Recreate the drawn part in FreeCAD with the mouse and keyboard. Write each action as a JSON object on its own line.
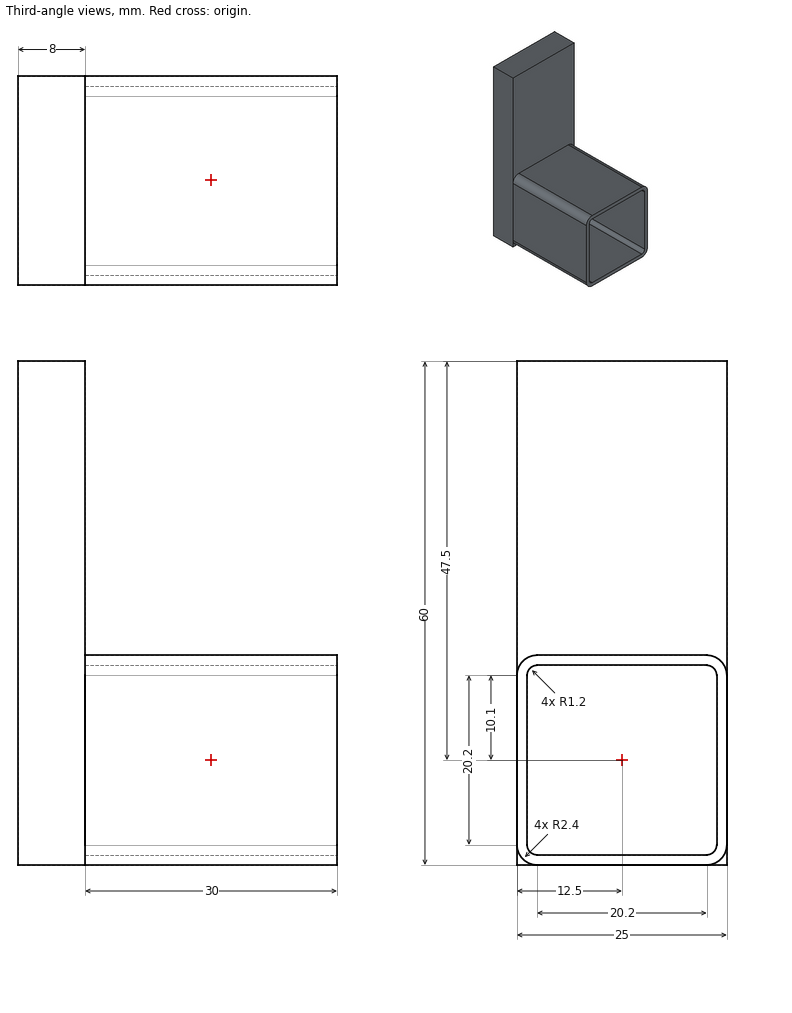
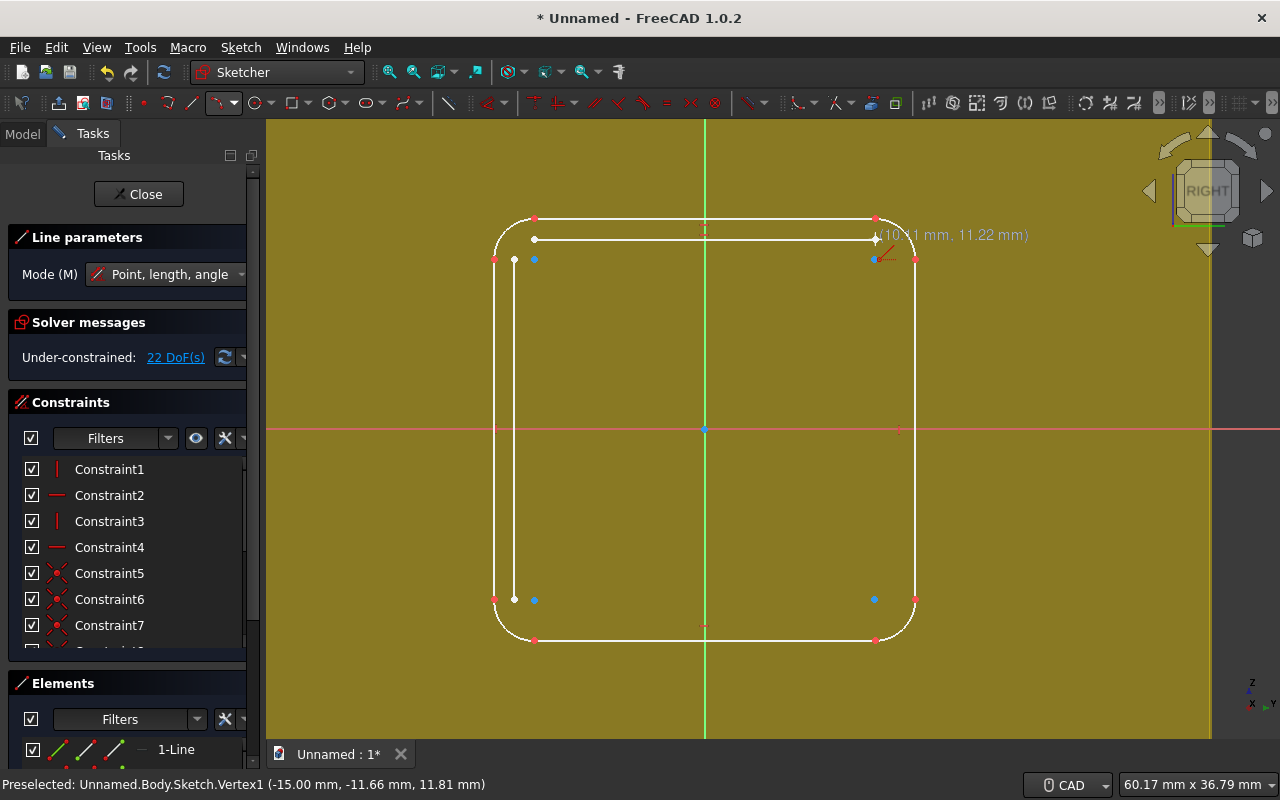
{"action": "left_click", "coordinate": [895, 259]}
{"action": "left_click", "coordinate": [895, 599]}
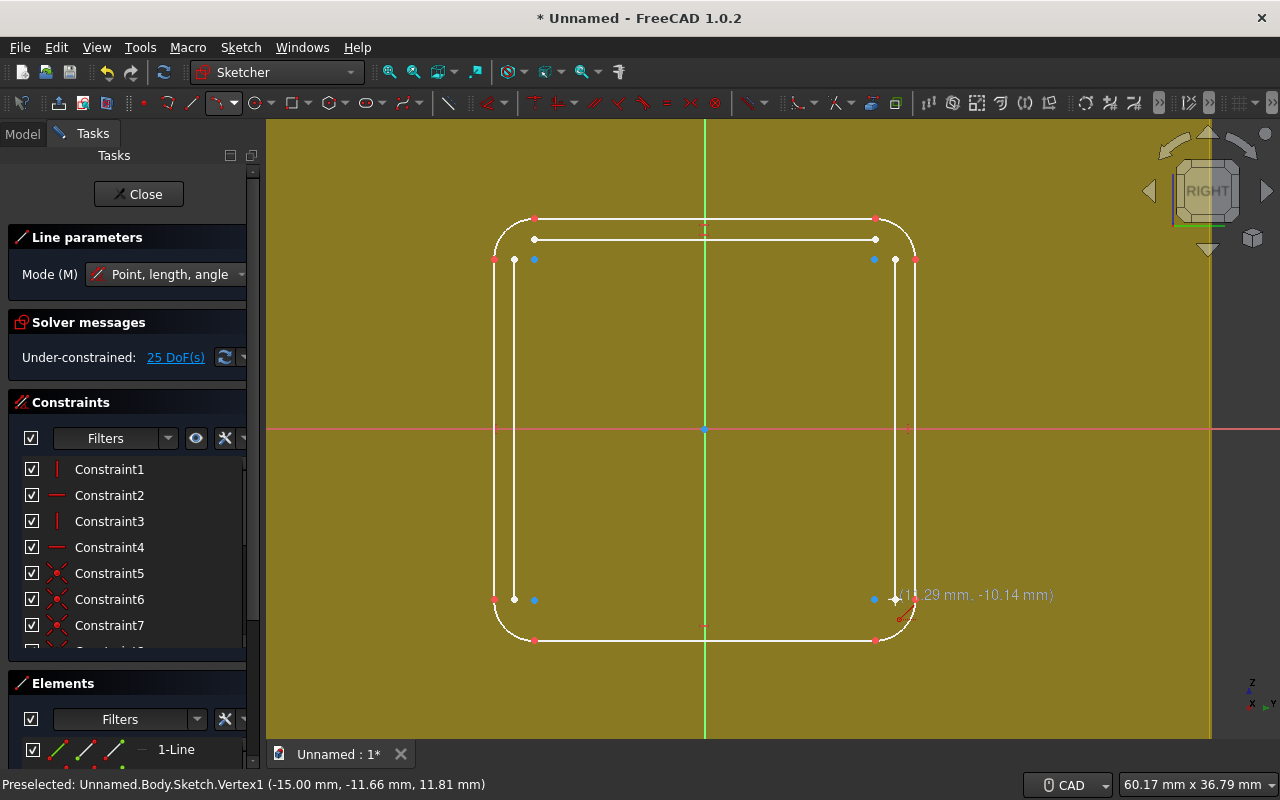
{"action": "left_click", "coordinate": [875, 620]}
{"action": "left_click", "coordinate": [534, 620]}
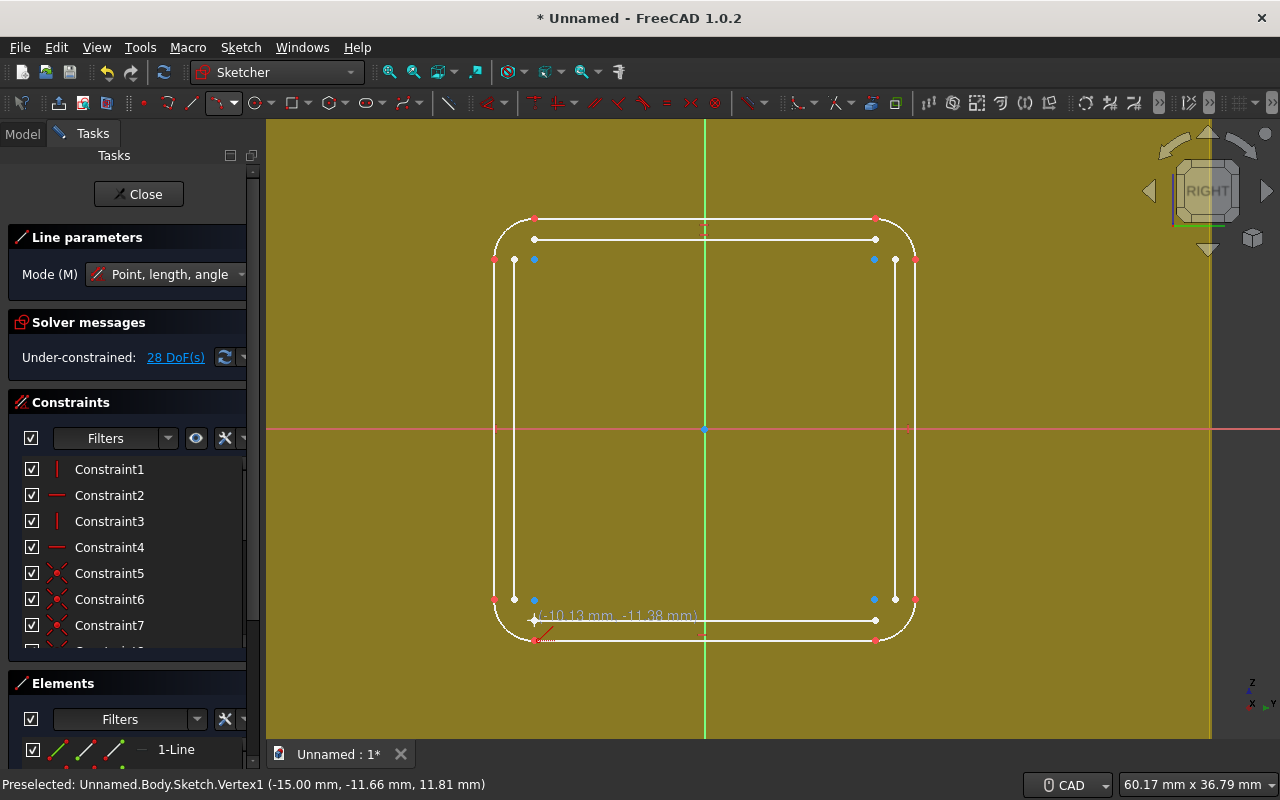
{"action": "key", "text": "g 3 a"}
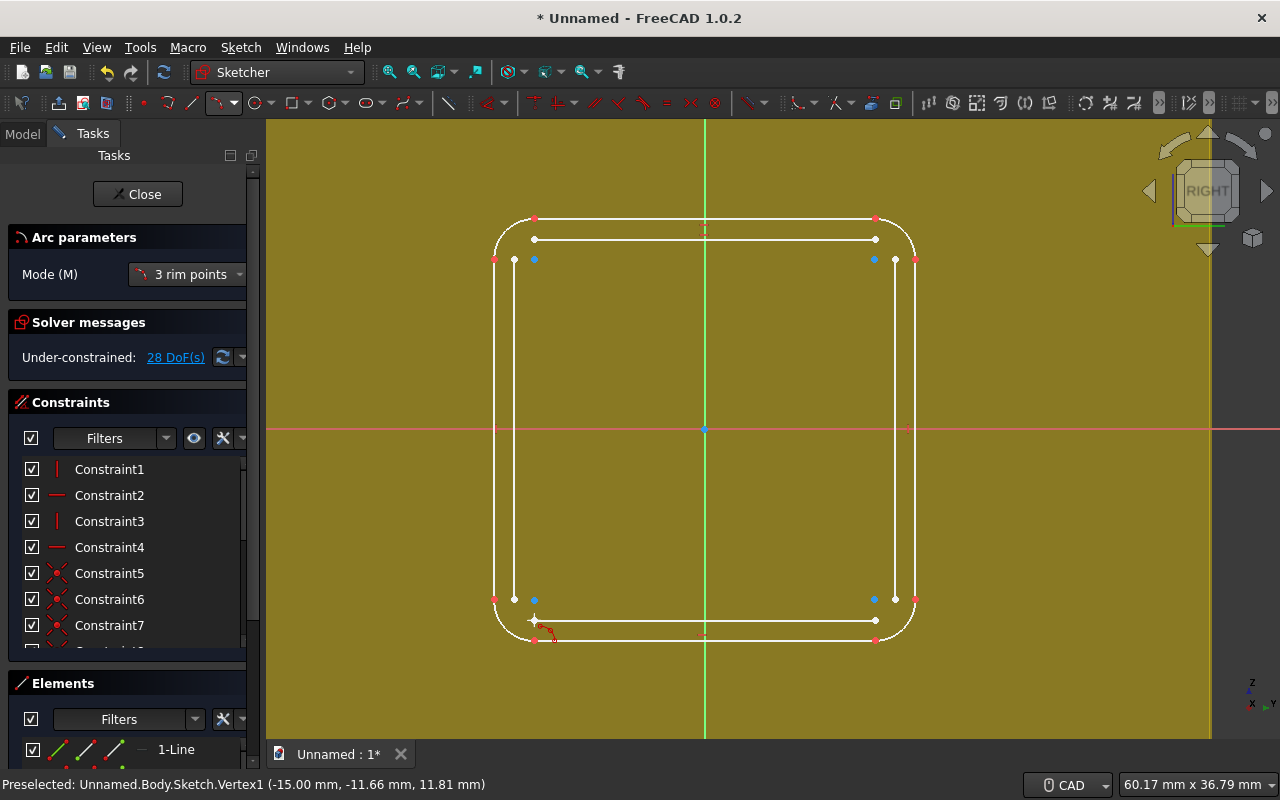
{"action": "left_click", "coordinate": [514, 260]}
{"action": "left_click", "coordinate": [534, 240]}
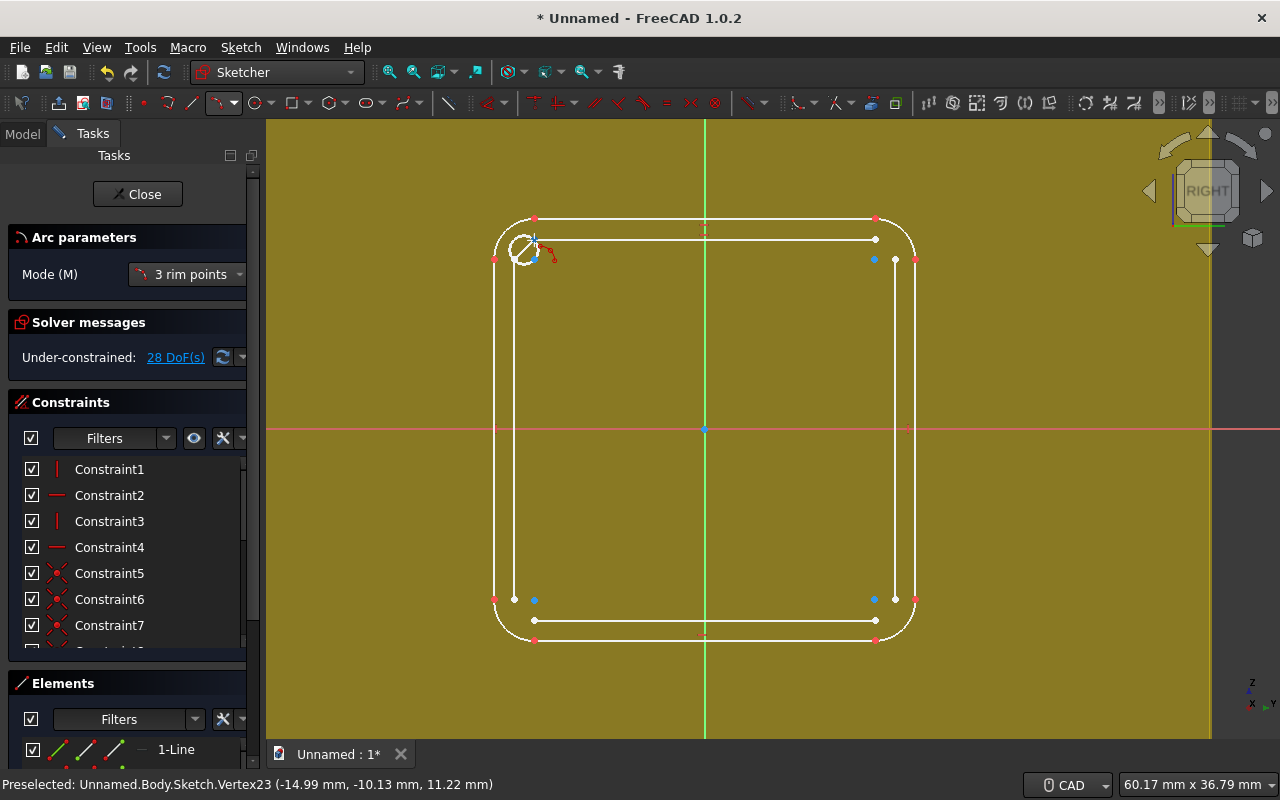
{"action": "scroll", "coordinate": [520, 245], "scroll_direction": "up", "scroll_amount": 5}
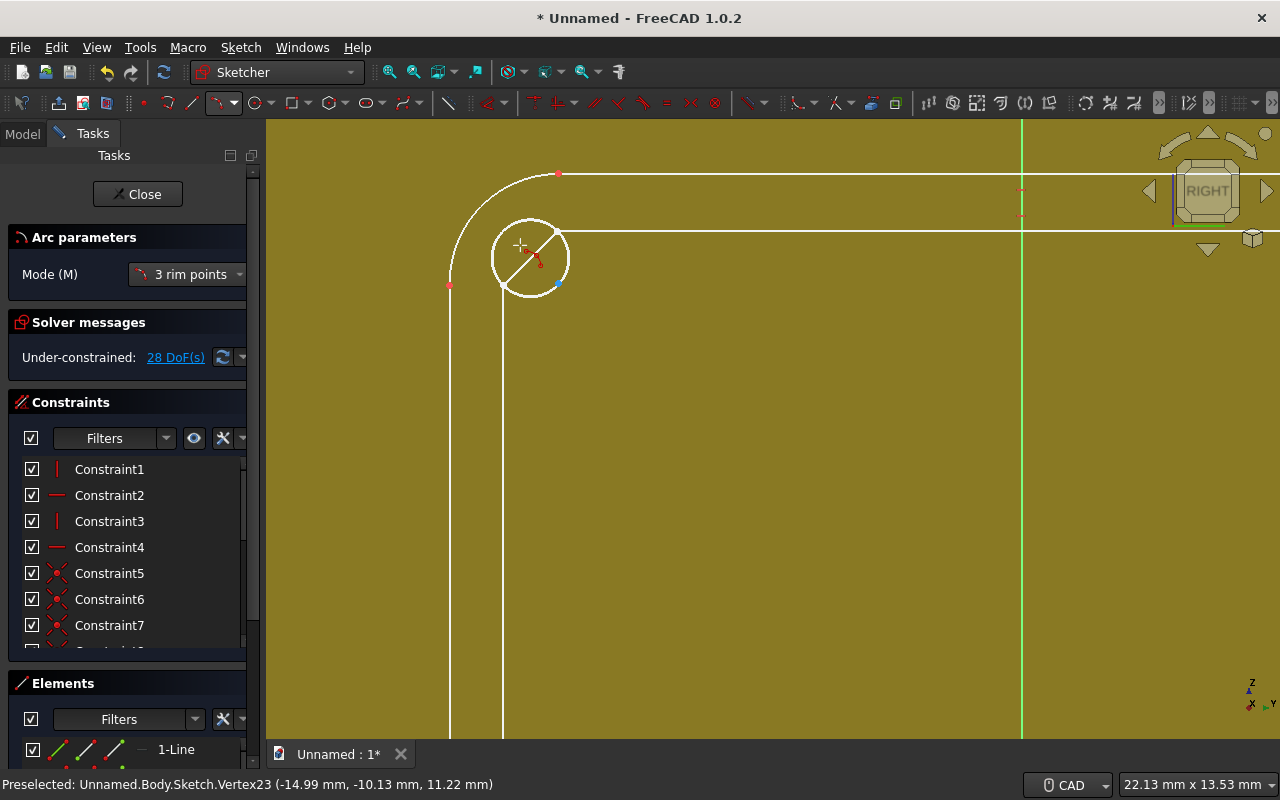
{"action": "left_click", "coordinate": [520, 244]}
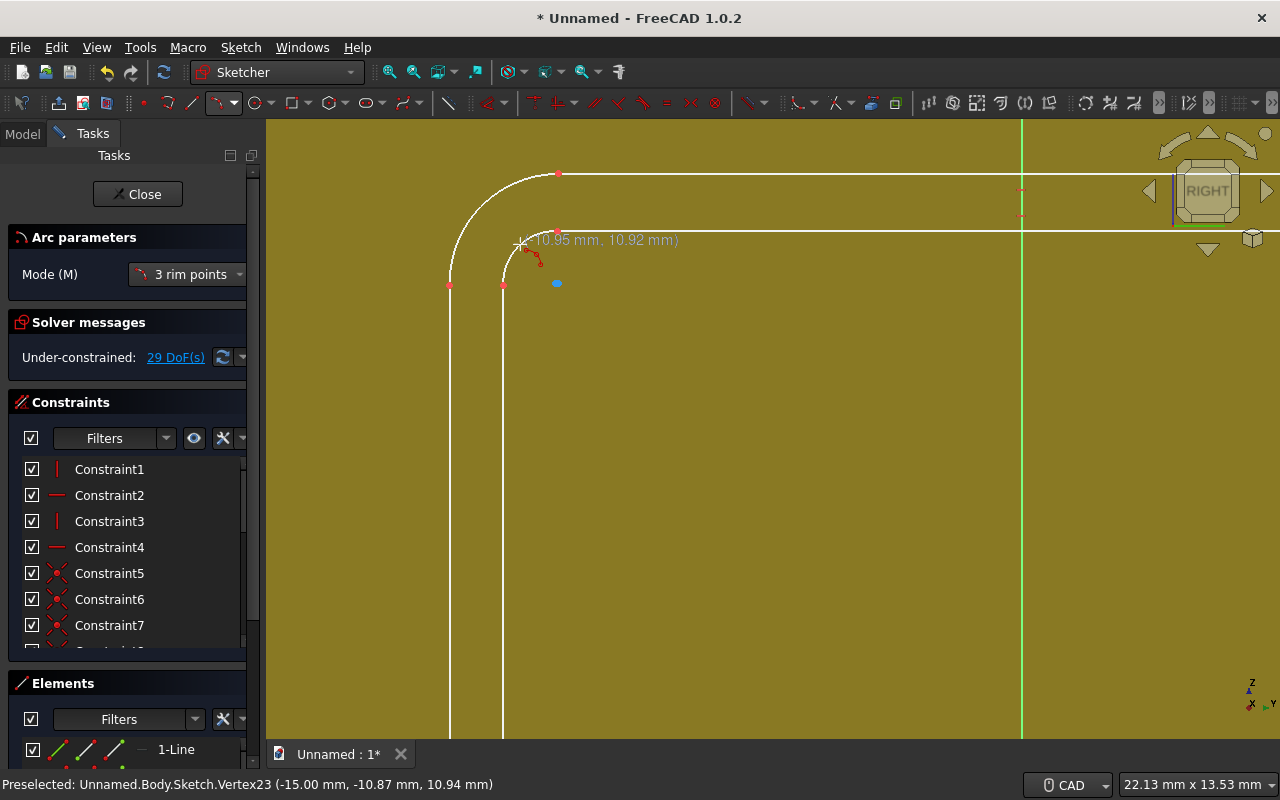
{"action": "scroll", "coordinate": [520, 245], "scroll_direction": "down", "scroll_amount": 5}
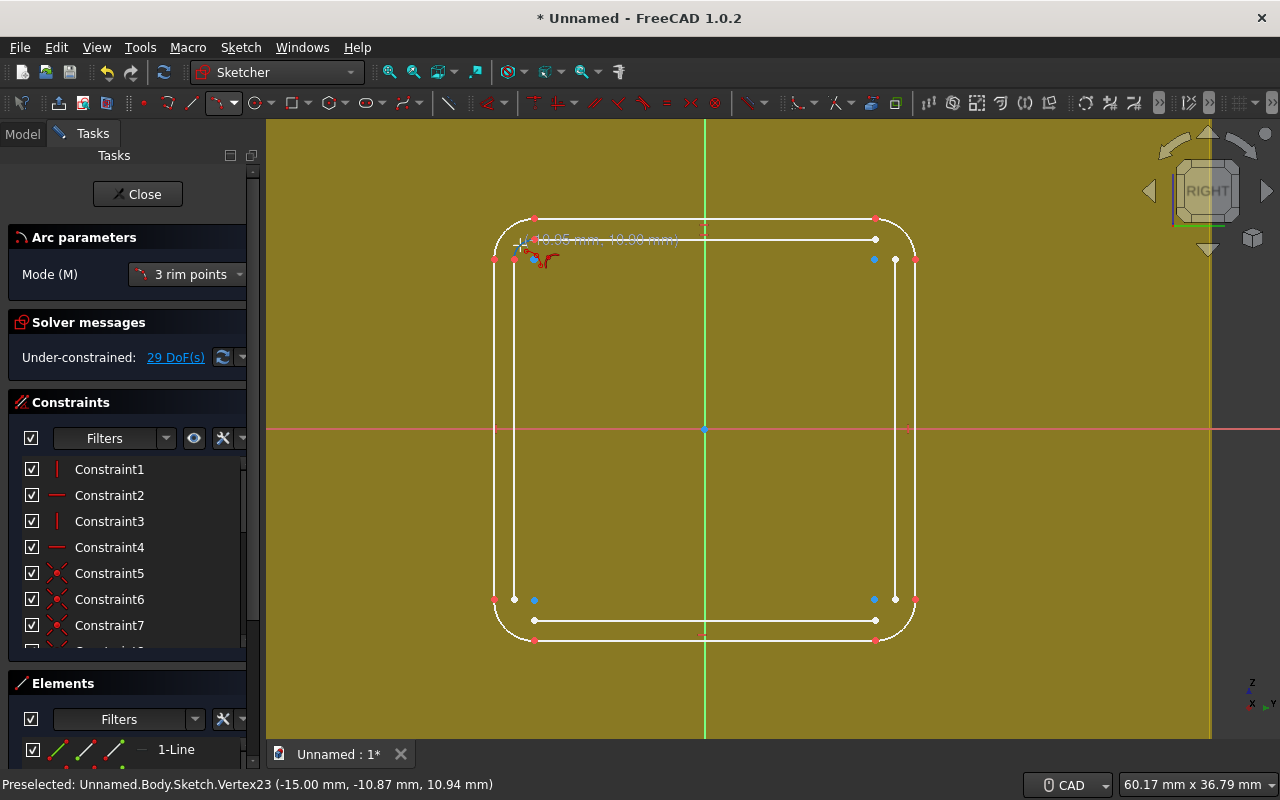
{"action": "left_click", "coordinate": [875, 240]}
{"action": "left_click", "coordinate": [895, 260]}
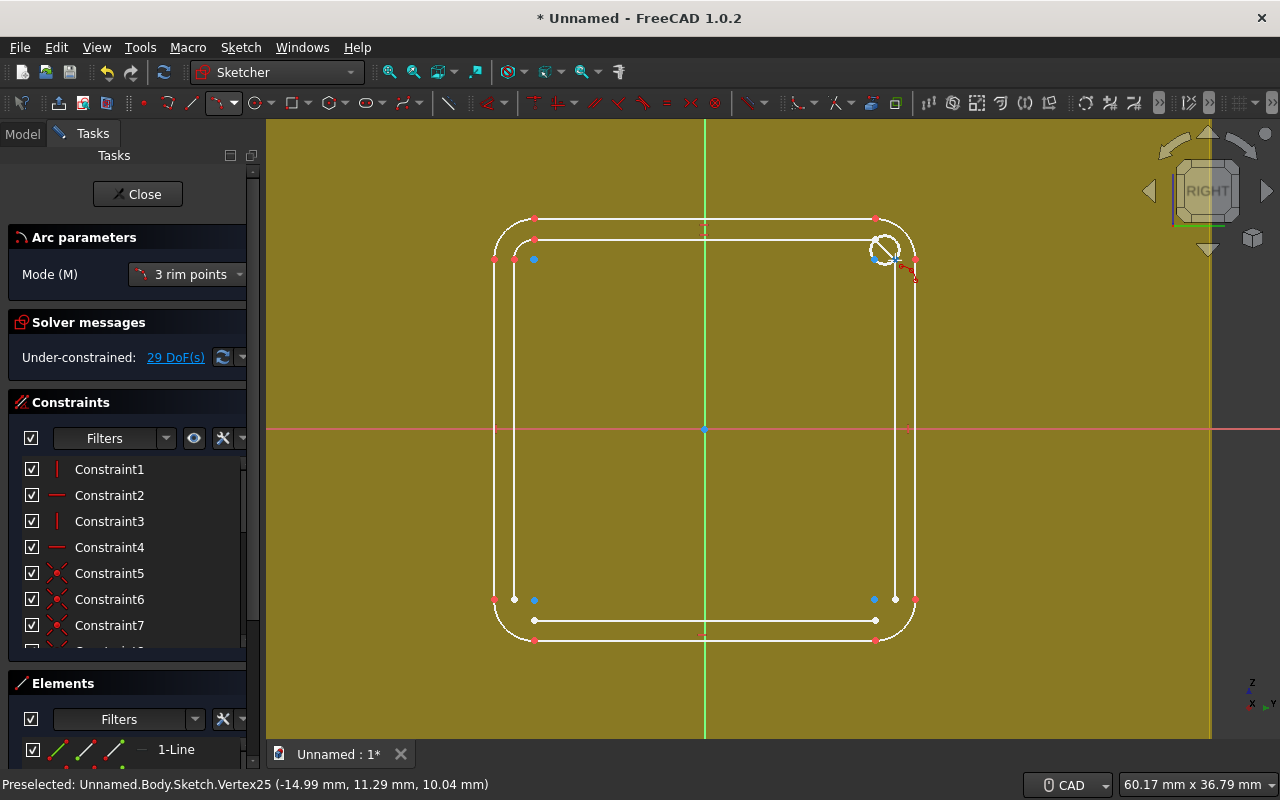
{"action": "scroll", "coordinate": [889, 245], "scroll_direction": "up", "scroll_amount": 5}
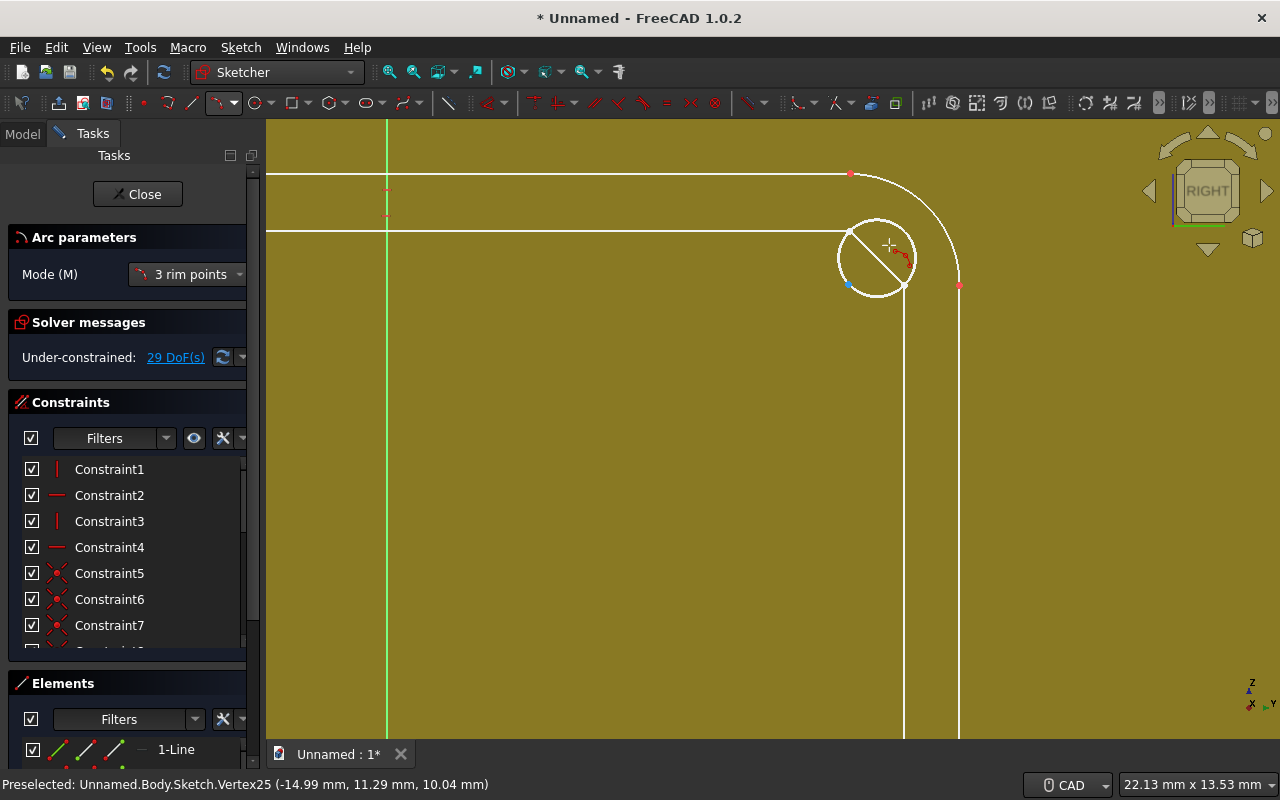
{"action": "left_click", "coordinate": [888, 244]}